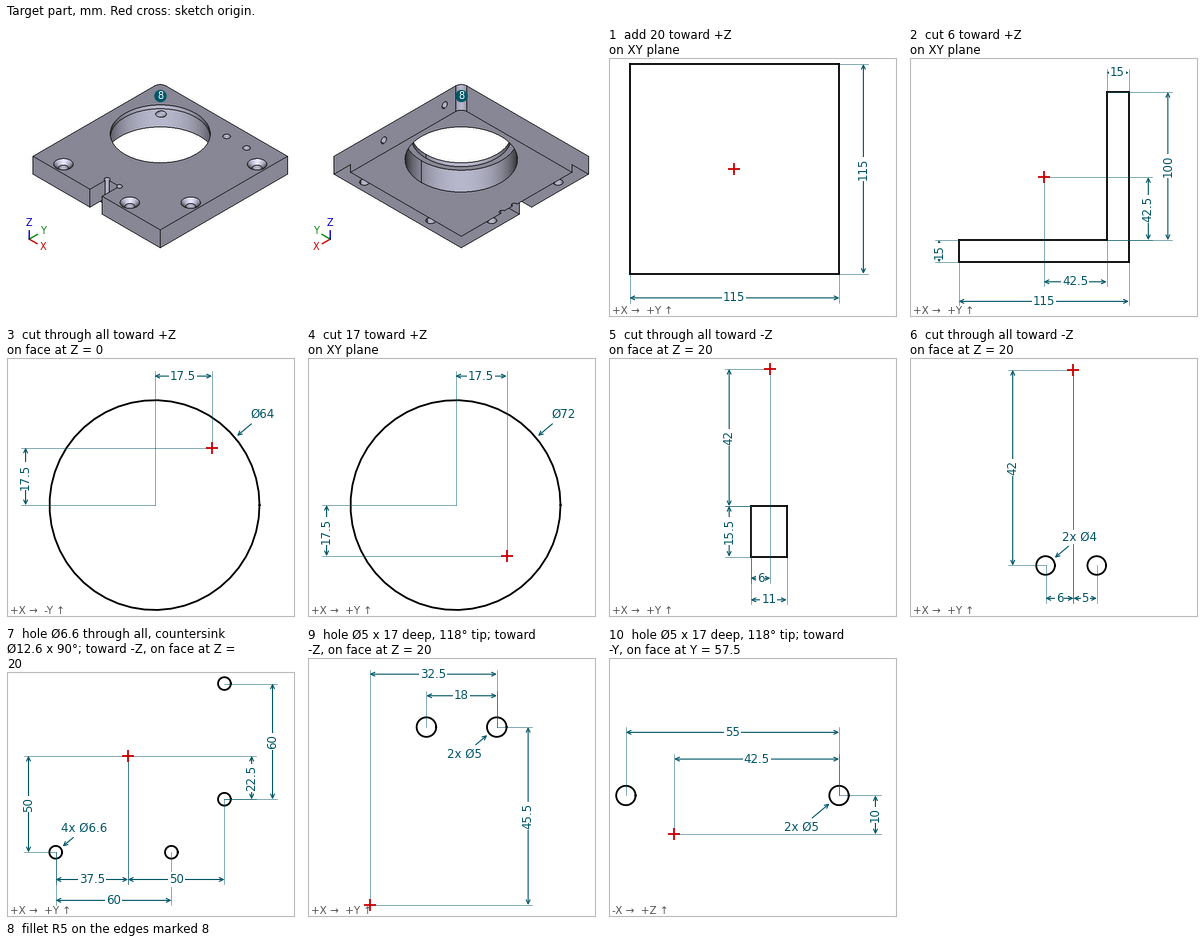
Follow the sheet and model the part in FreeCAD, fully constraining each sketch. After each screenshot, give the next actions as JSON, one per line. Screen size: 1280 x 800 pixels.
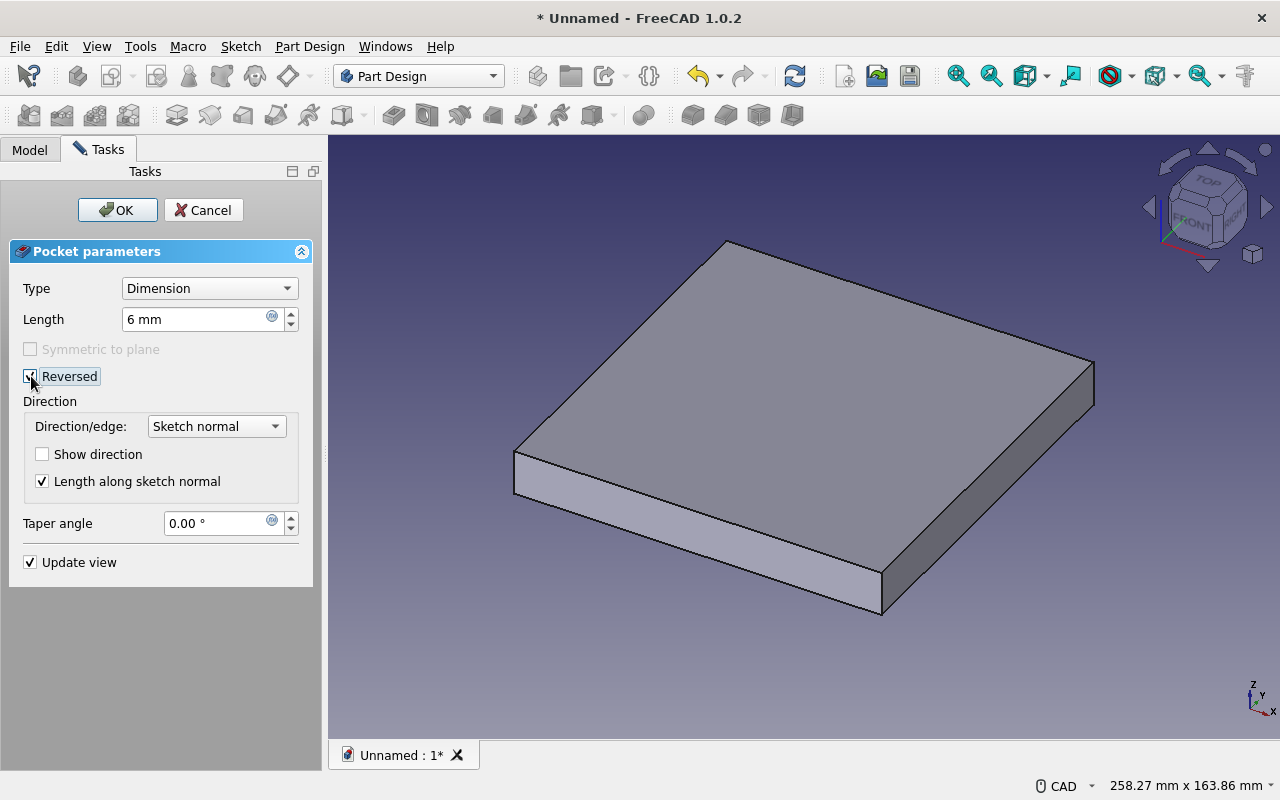
{"action": "left_click", "coordinate": [118, 210]}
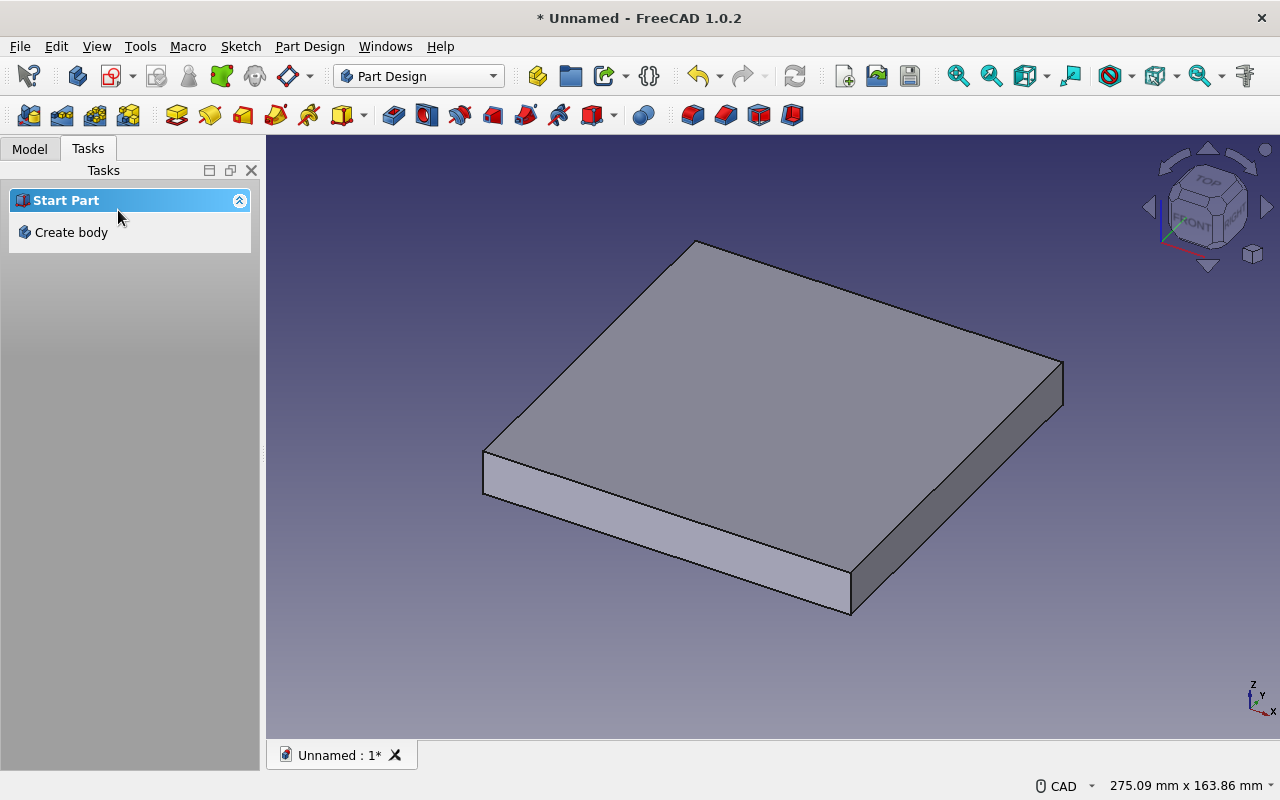
{"action": "key", "text": "5"}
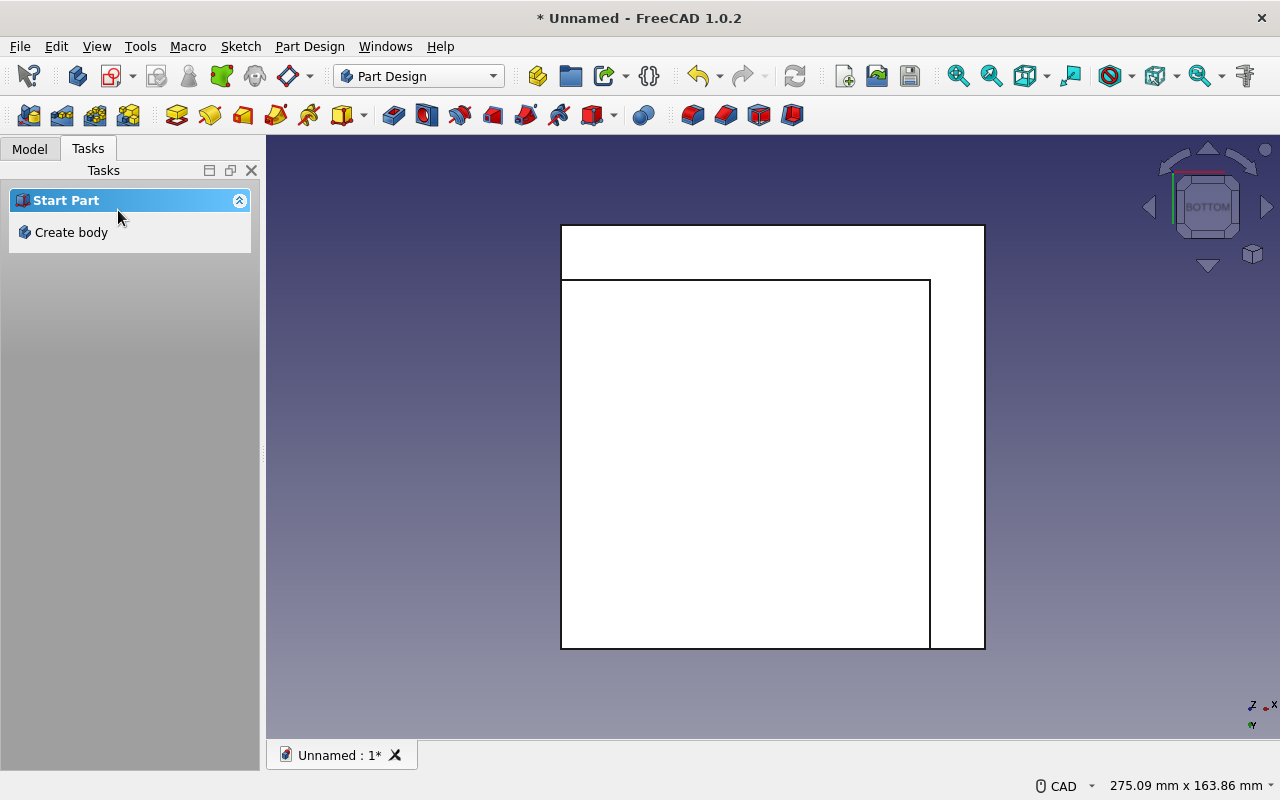
{"action": "left_click", "coordinate": [745, 464]}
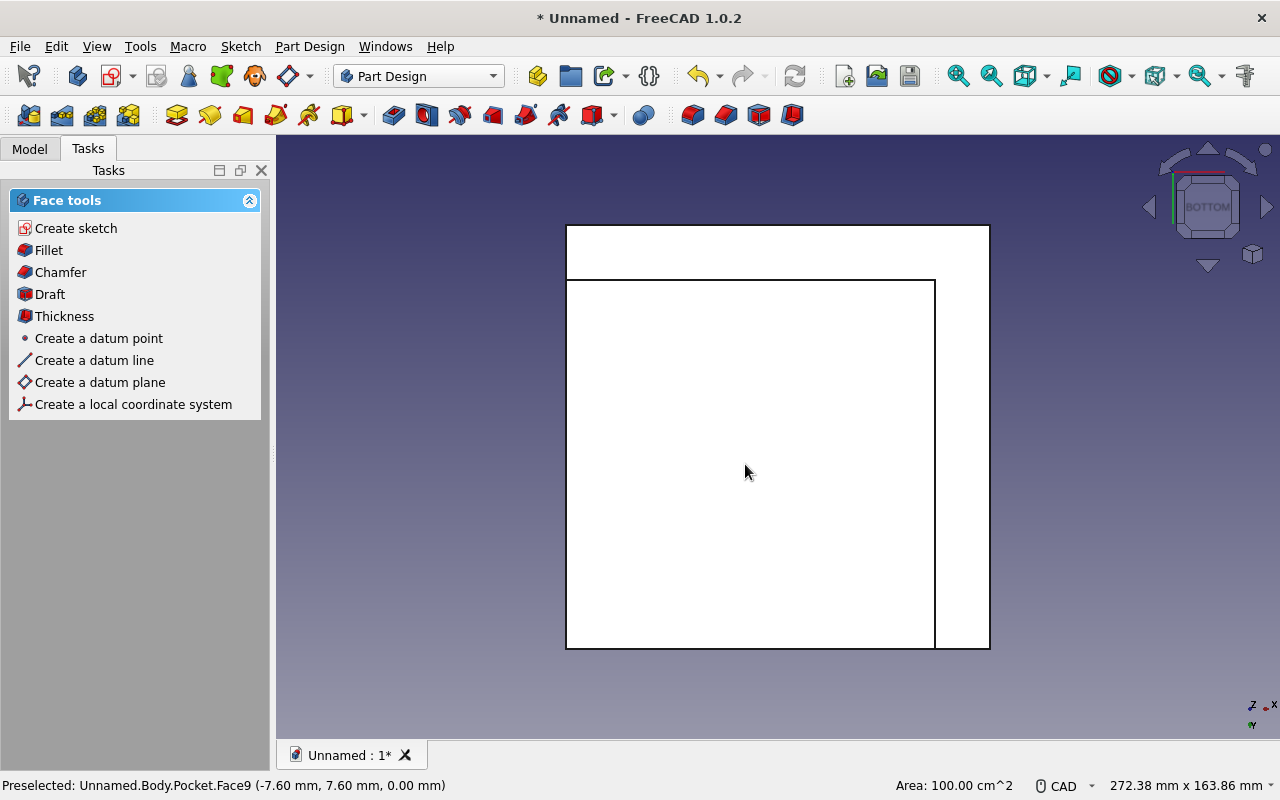
{"action": "left_click", "coordinate": [110, 76]}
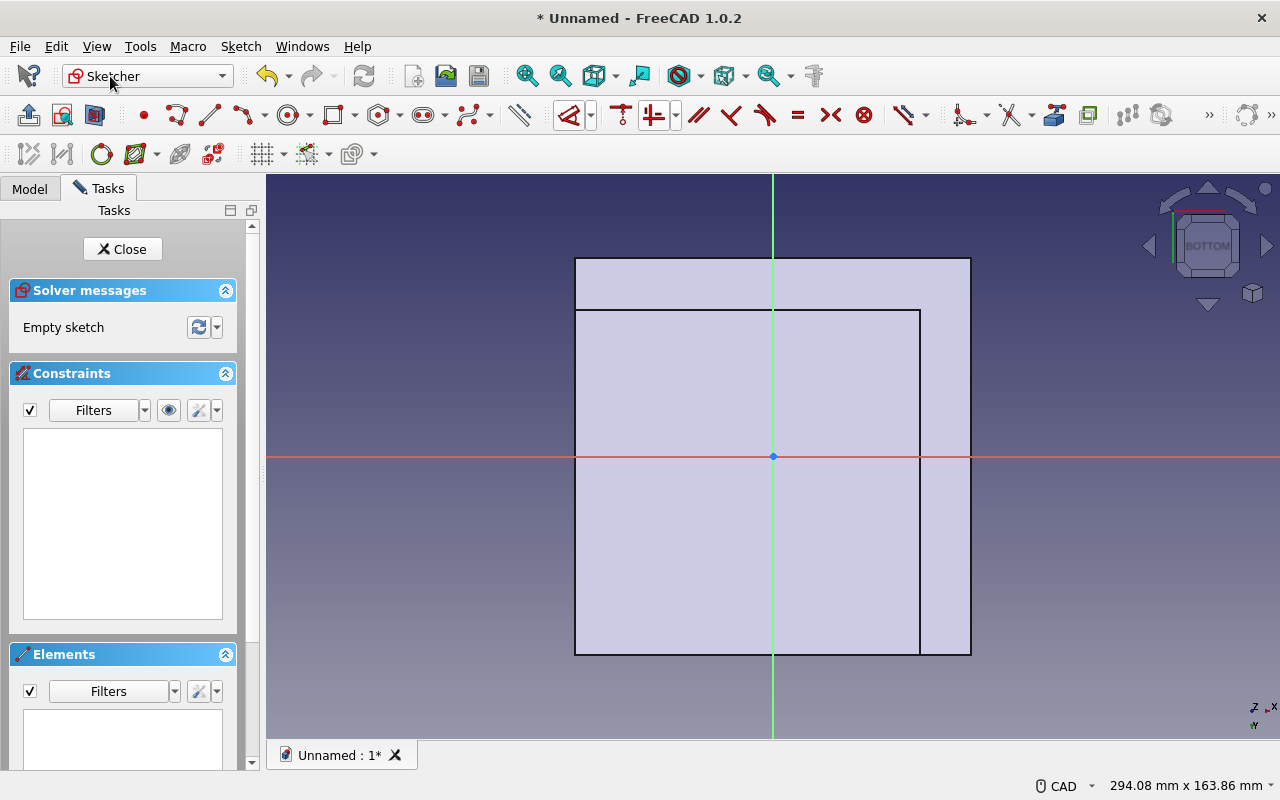
{"action": "scroll", "coordinate": [729, 640], "scroll_direction": "up", "scroll_amount": 2}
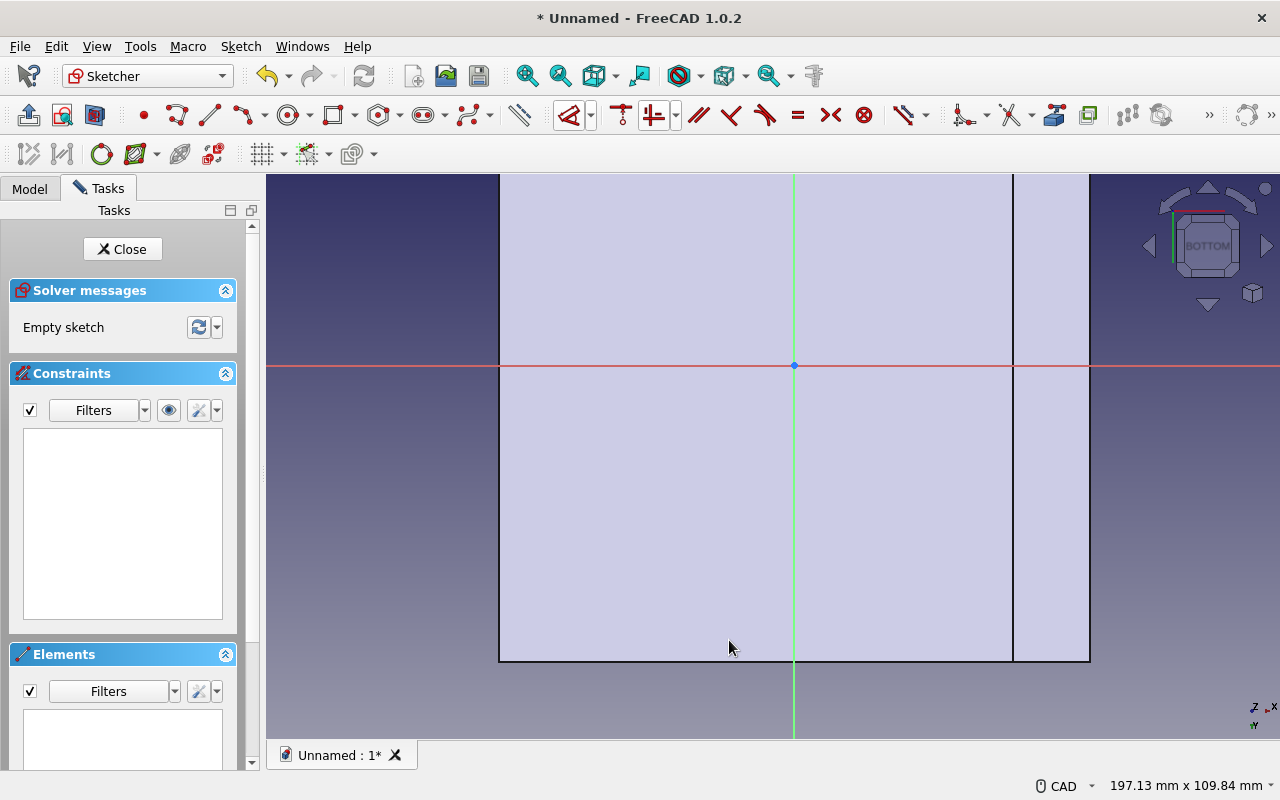
{"action": "left_click", "coordinate": [288, 116]}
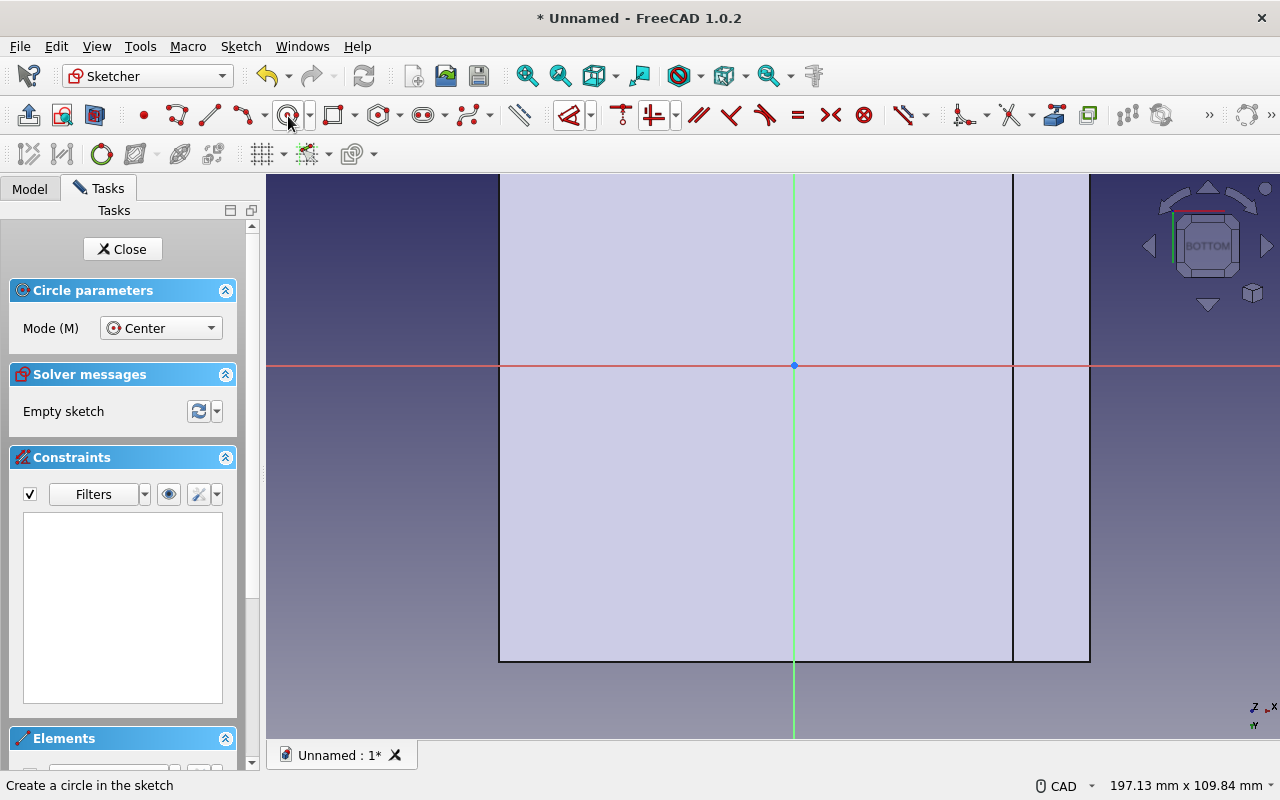
{"action": "left_click", "coordinate": [704, 456]}
{"action": "left_click", "coordinate": [821, 339]}
{"action": "key", "text": "Escape"}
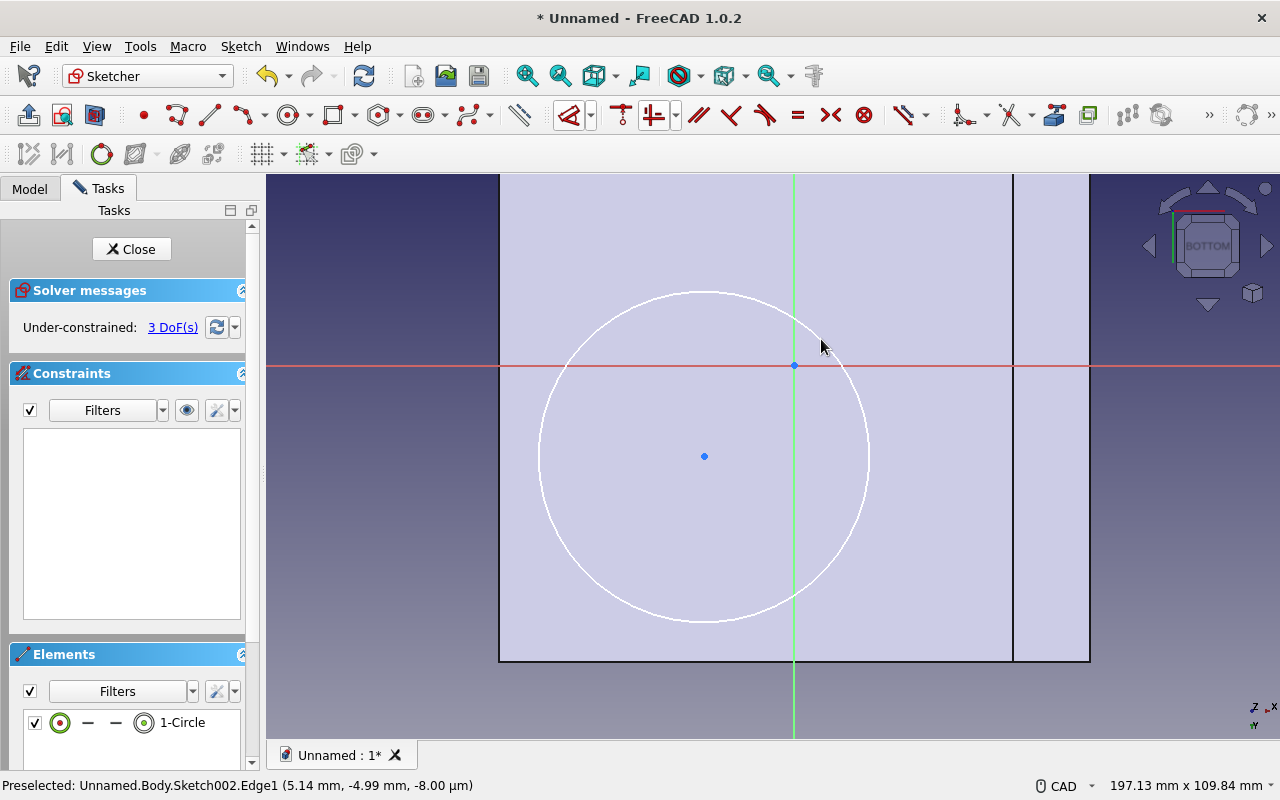
{"action": "left_click", "coordinate": [821, 340]}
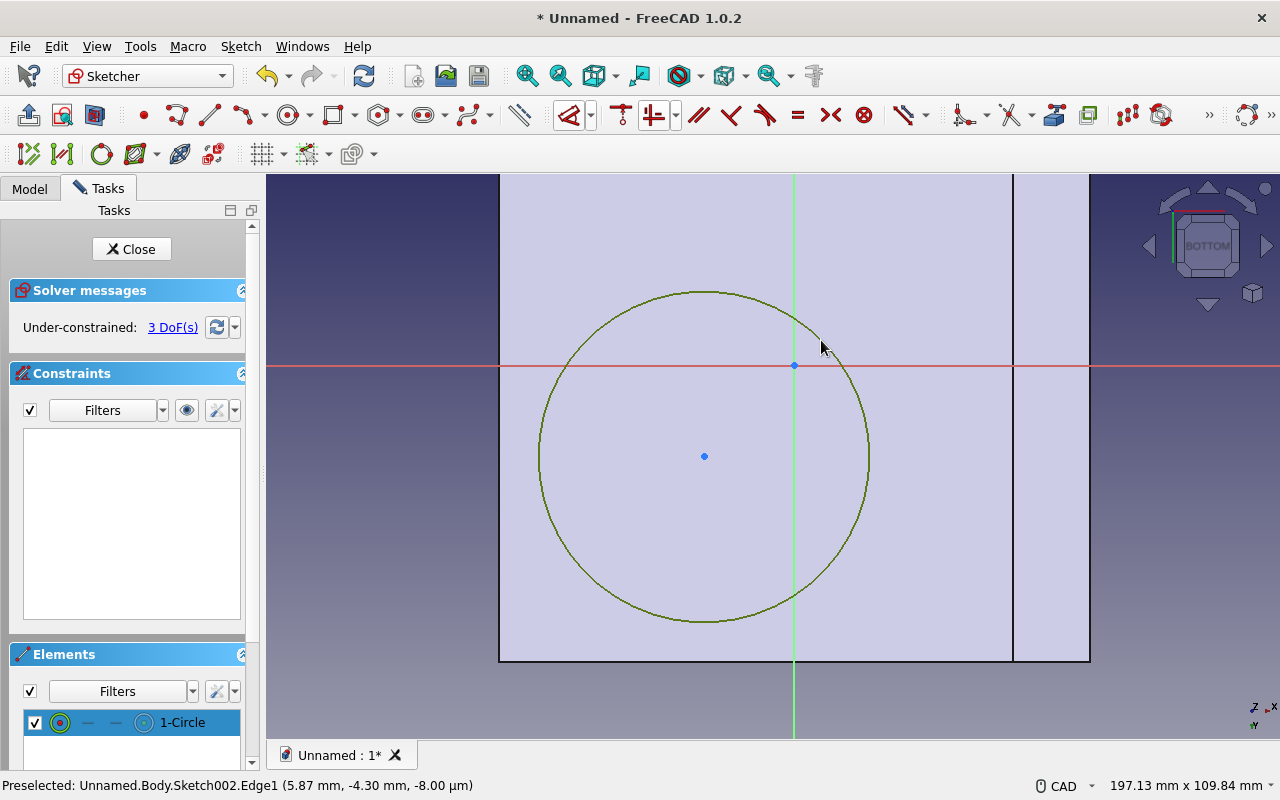
{"action": "key", "text": "k o"}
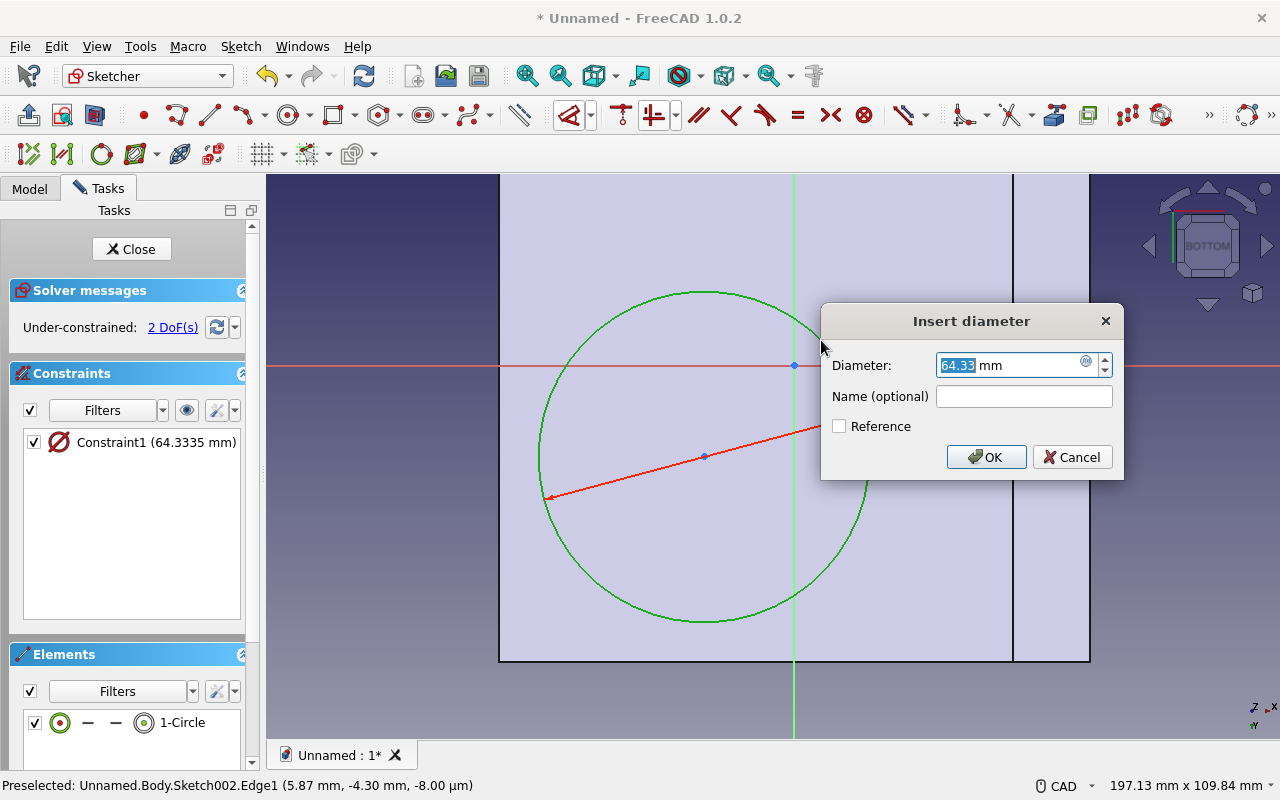
{"action": "type", "text": "64"}
{"action": "key", "text": "Return"}